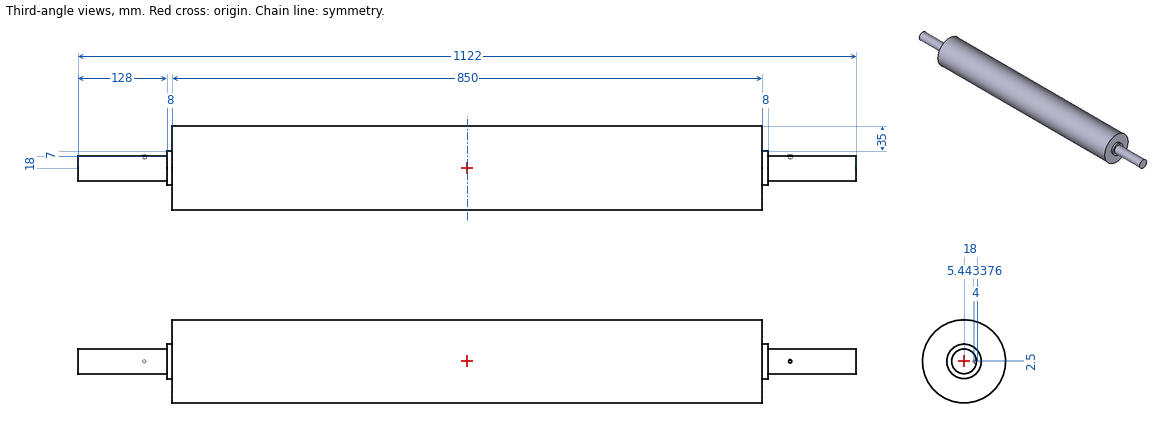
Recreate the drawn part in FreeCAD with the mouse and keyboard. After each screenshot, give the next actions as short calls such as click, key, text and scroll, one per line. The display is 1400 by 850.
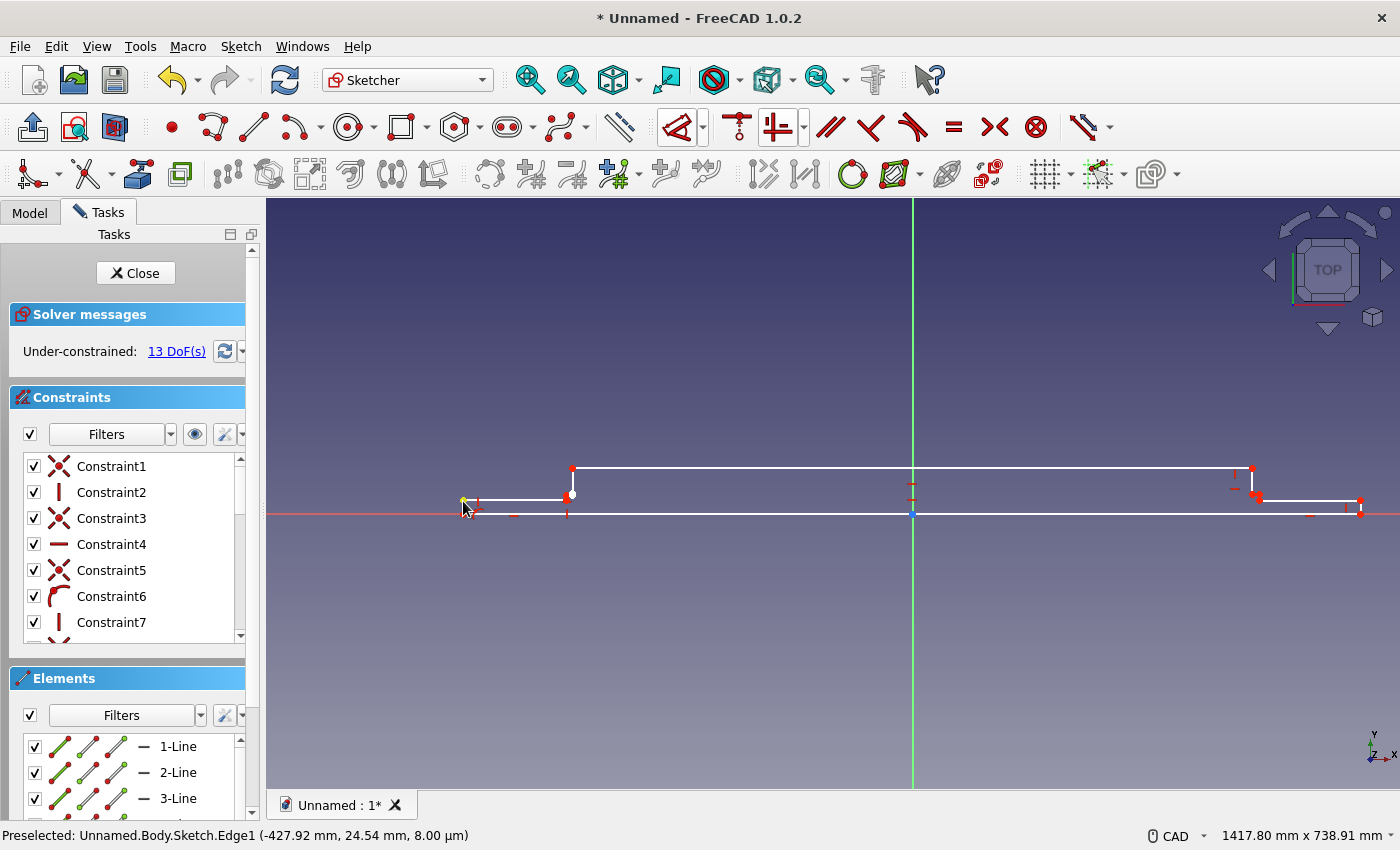
click(464, 500)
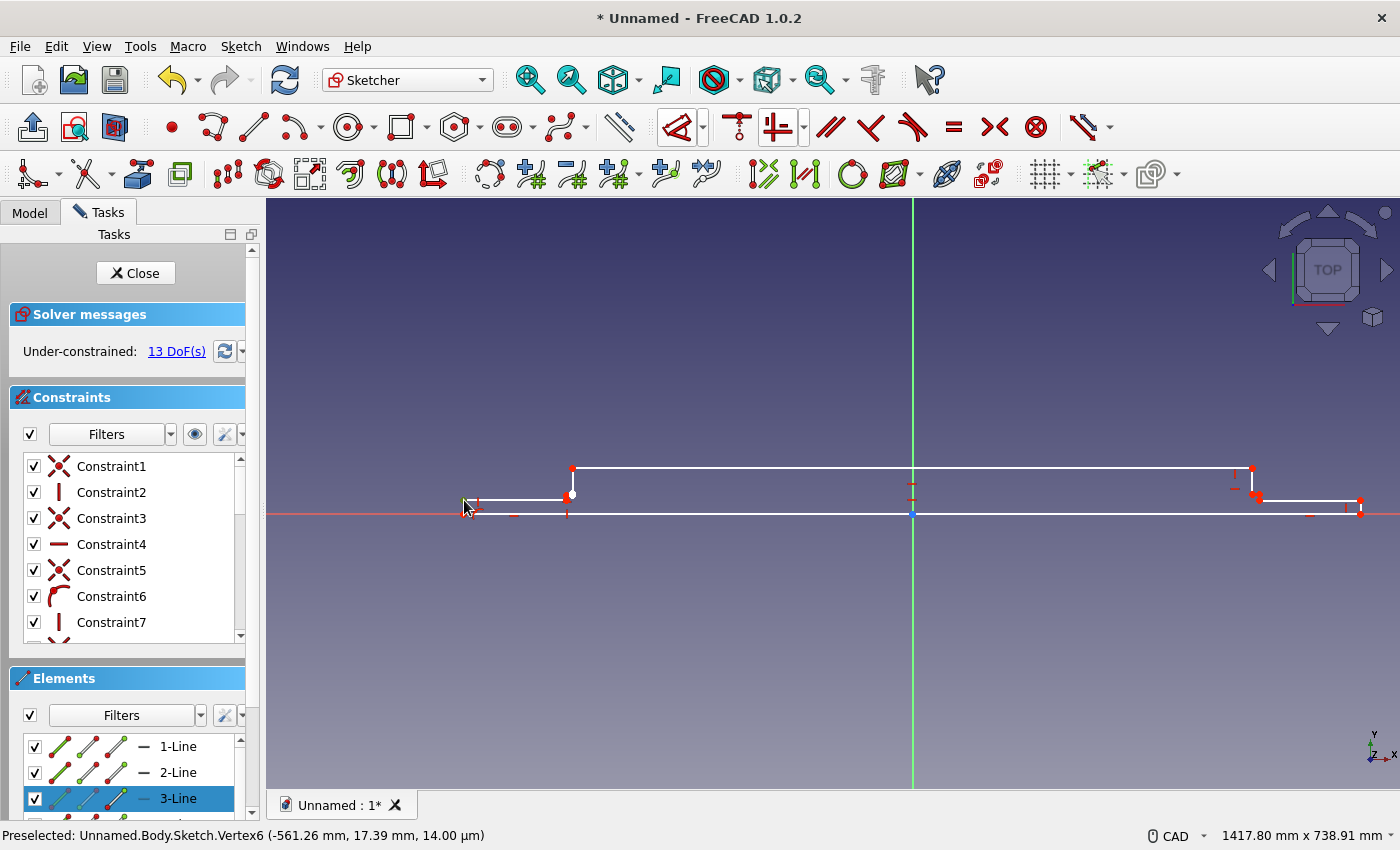
scroll(463, 500, down, 2)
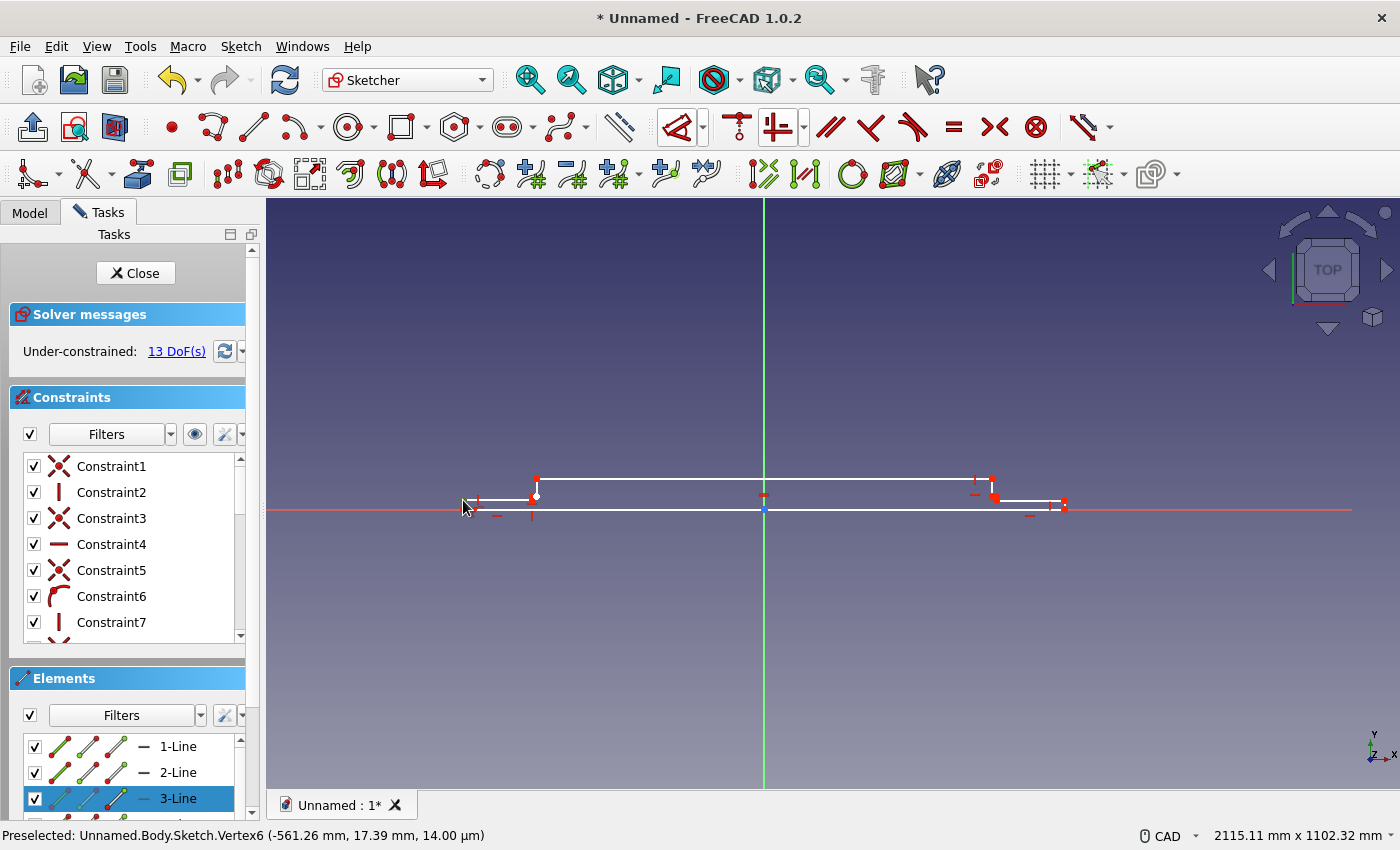
scroll(1065, 501, up, 2)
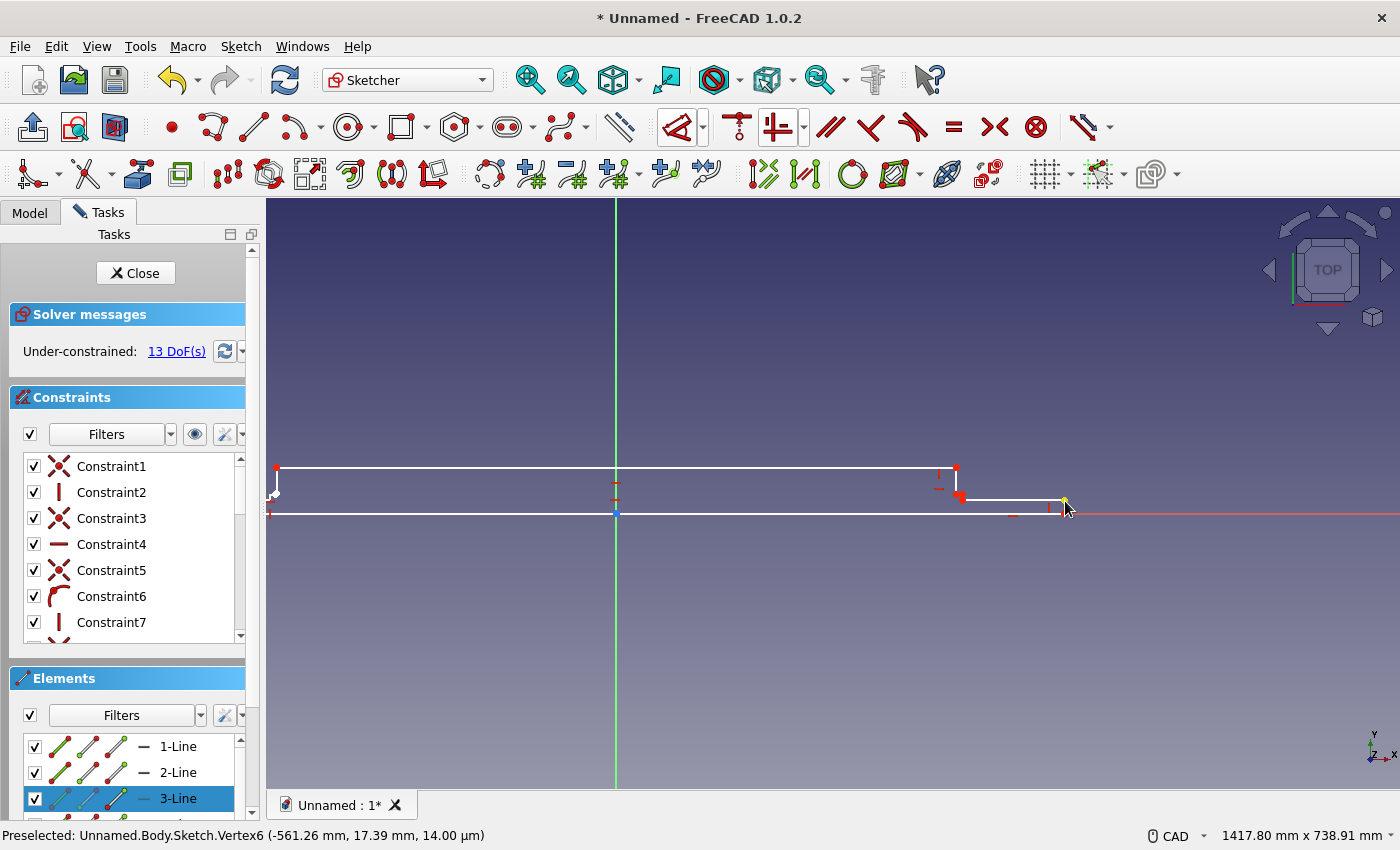
click(1065, 500)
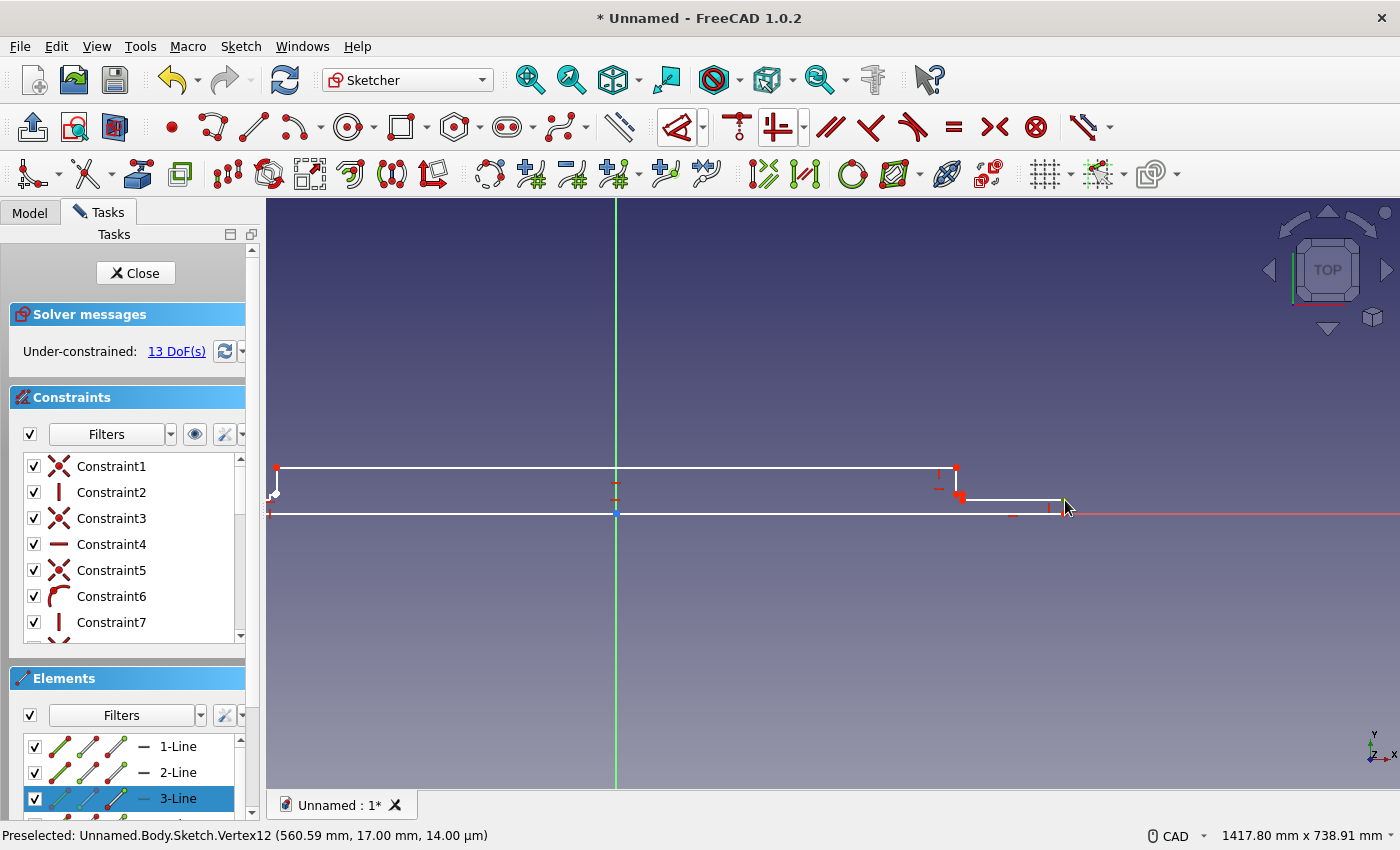
click(616, 723)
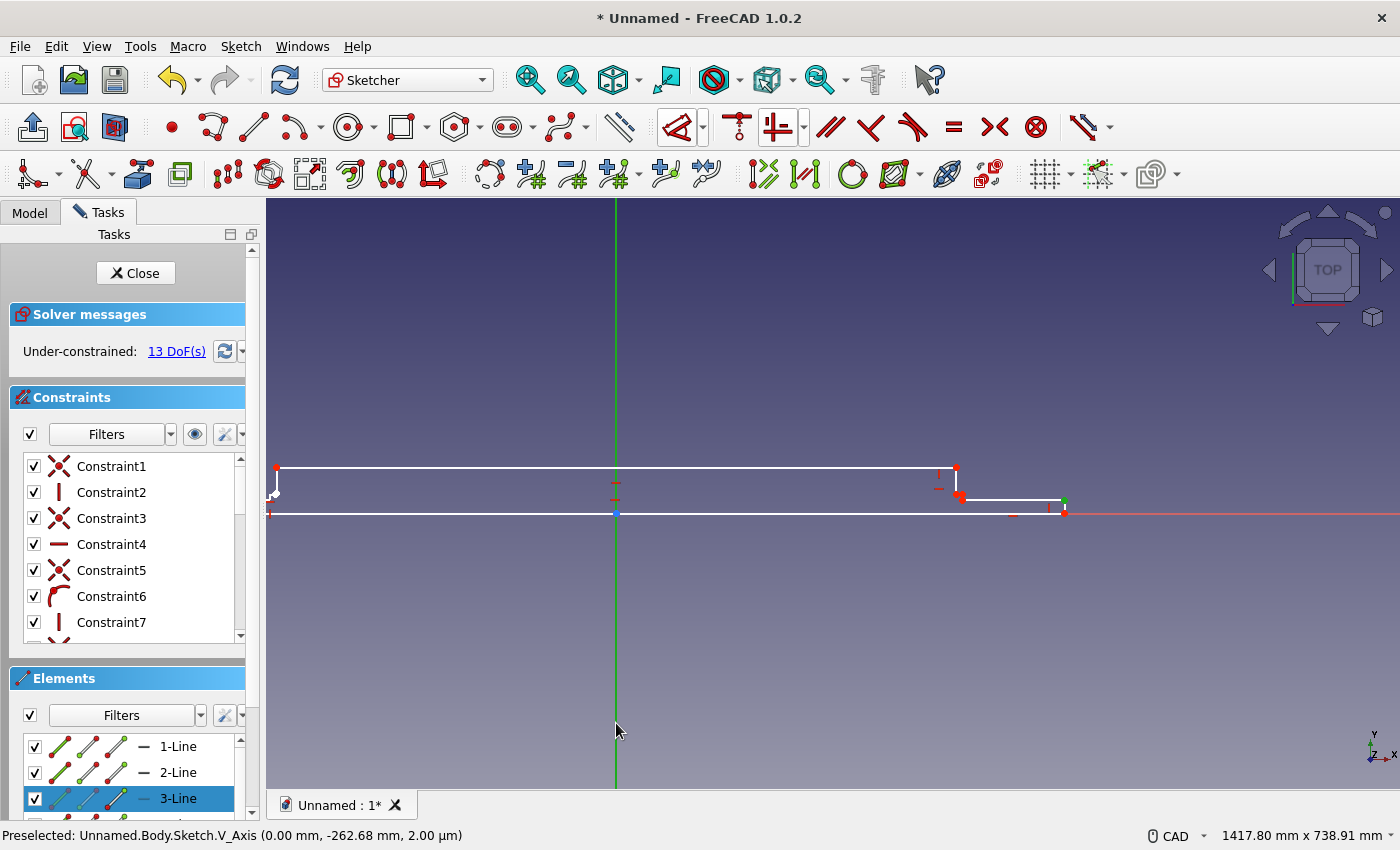
click(995, 128)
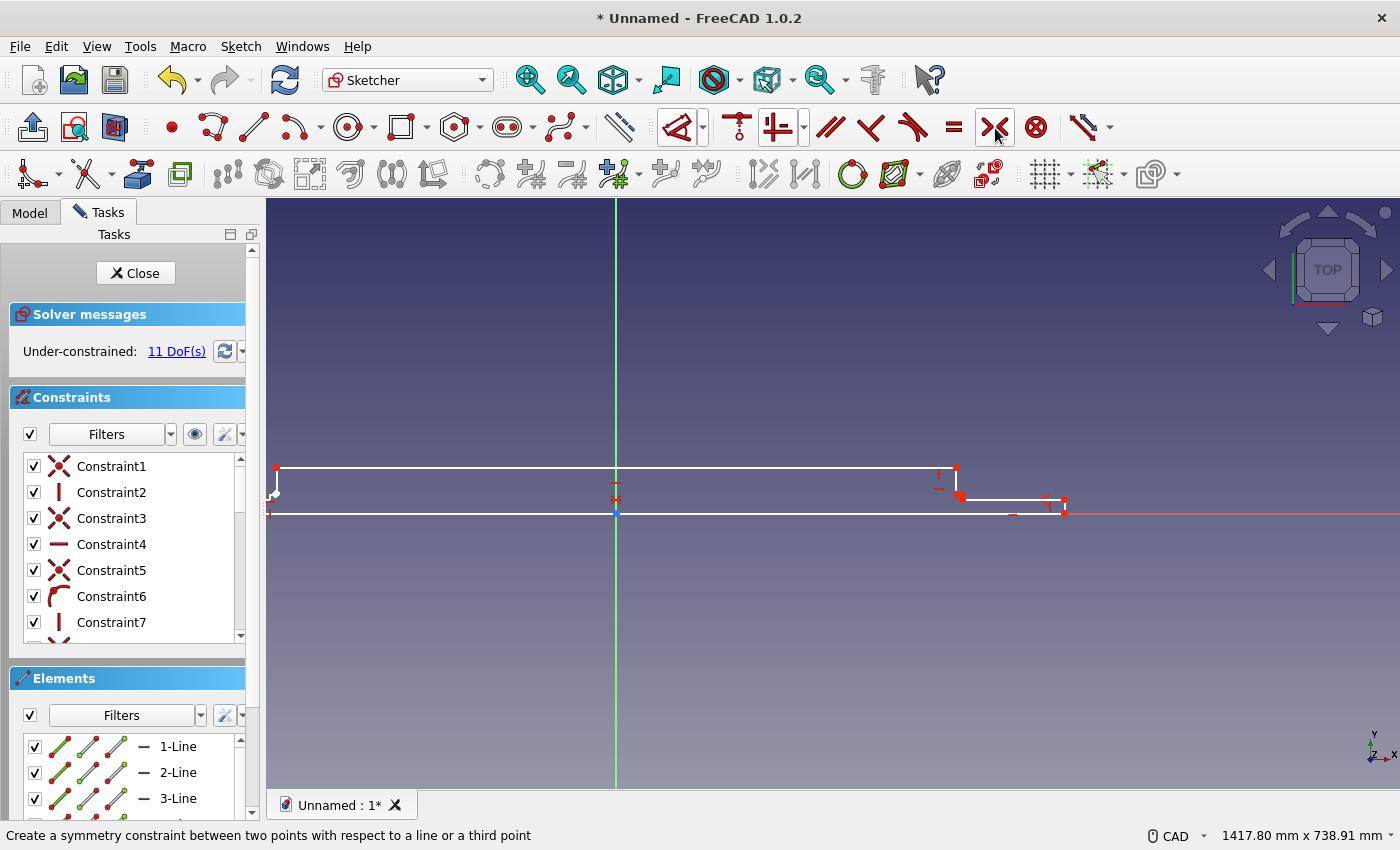
scroll(1066, 501, down, 2)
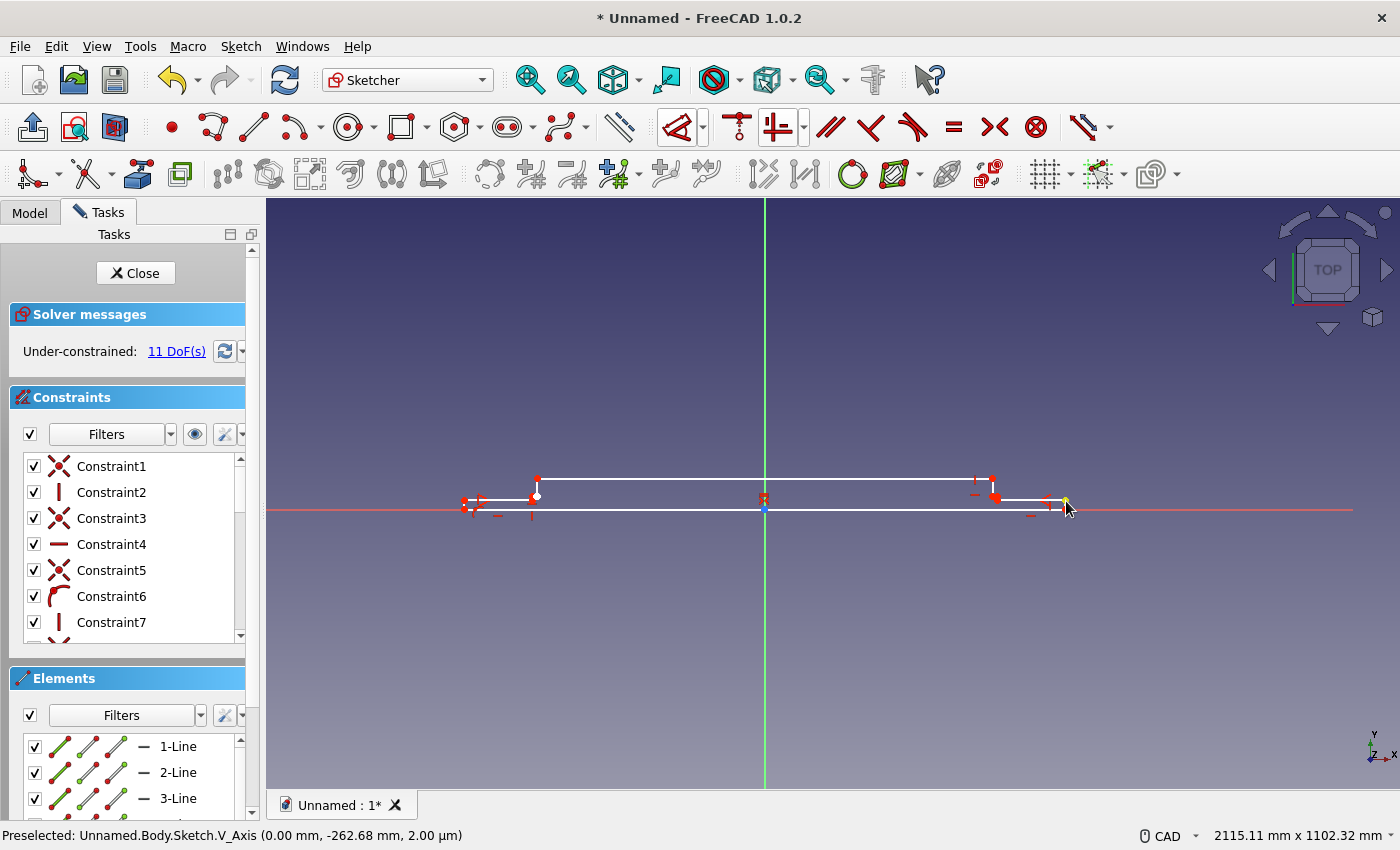
scroll(532, 497, up, 7)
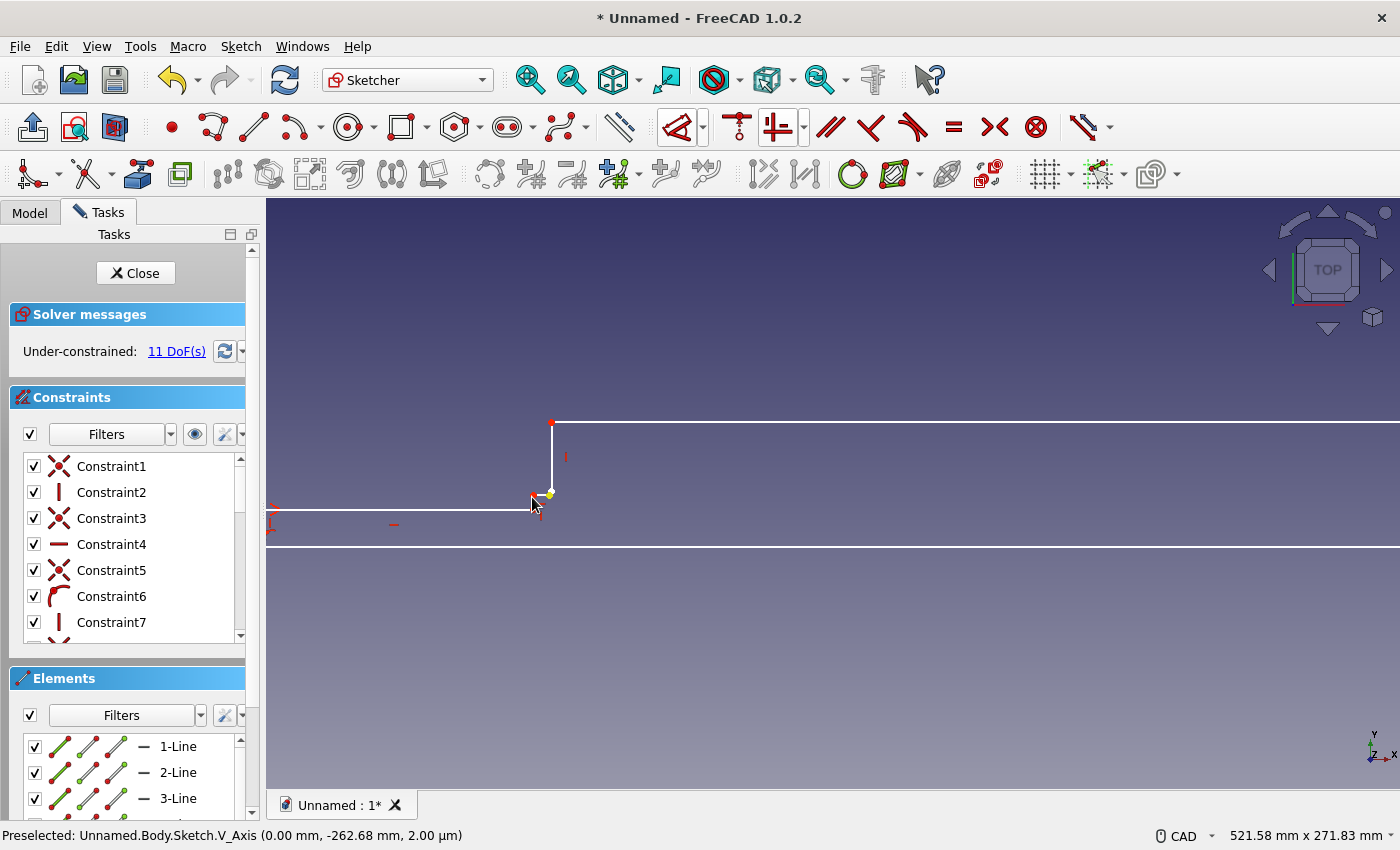
click(533, 495)